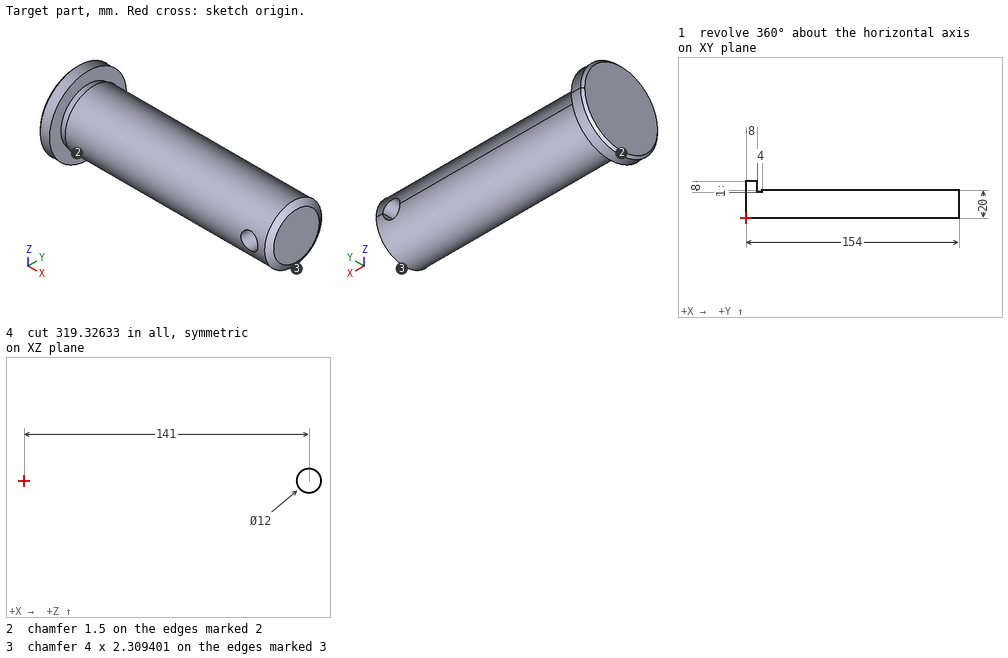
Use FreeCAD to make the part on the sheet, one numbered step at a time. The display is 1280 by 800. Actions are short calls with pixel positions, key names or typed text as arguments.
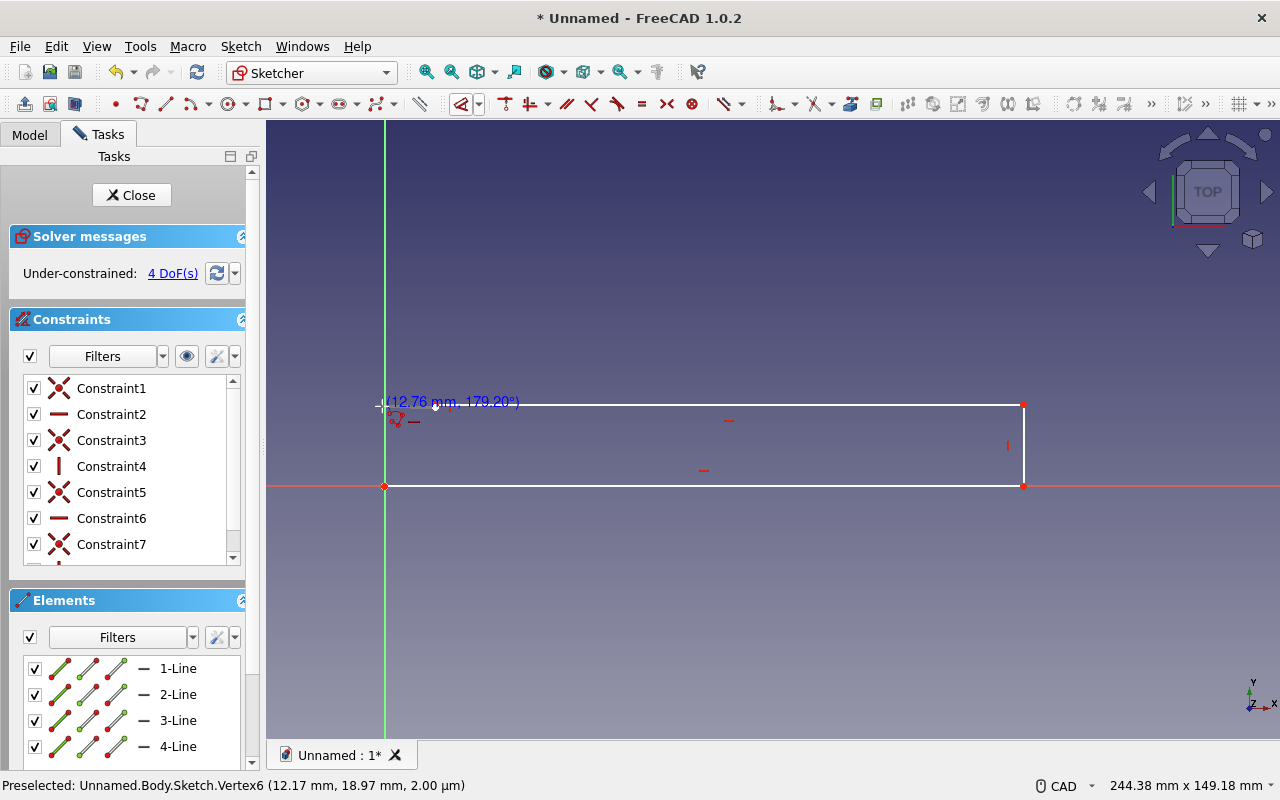
click(418, 407)
click(418, 374)
click(394, 374)
click(385, 486)
key(Escape)
key(Escape)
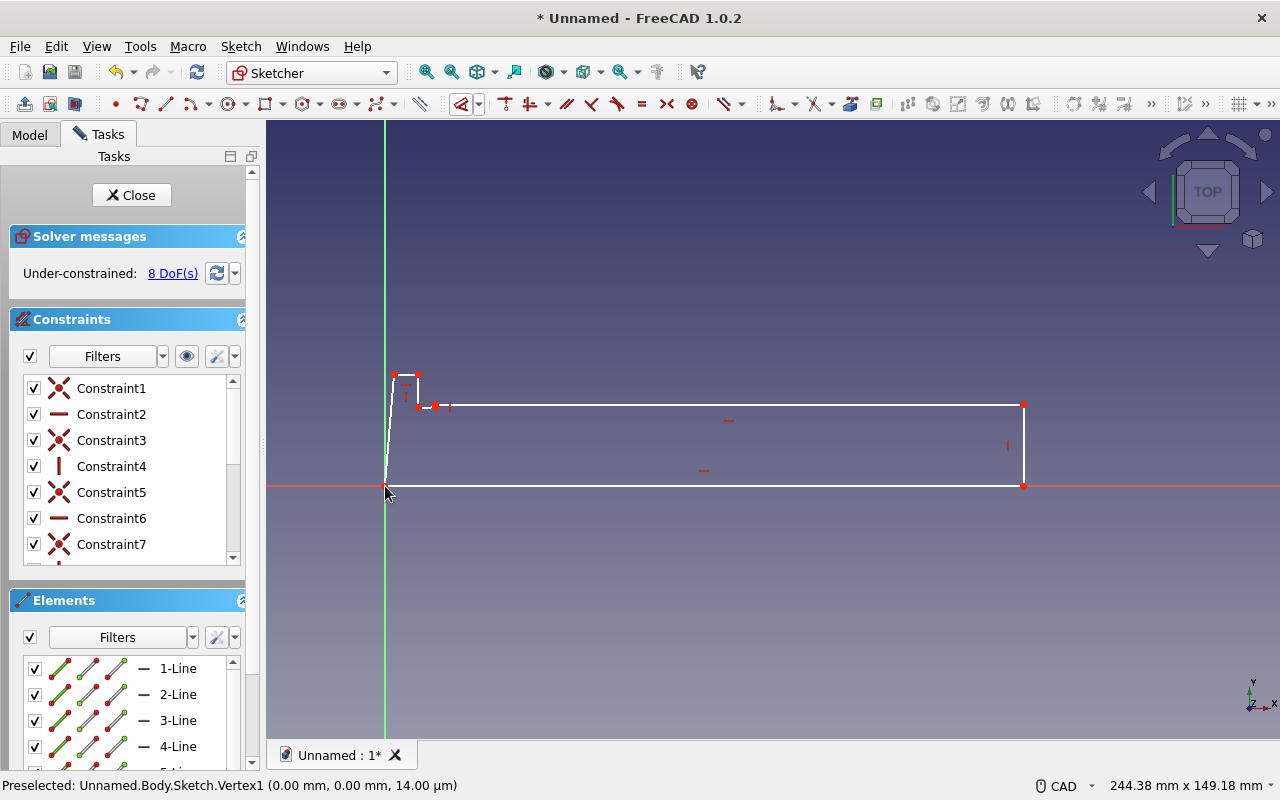
scroll(427, 408, up, 3)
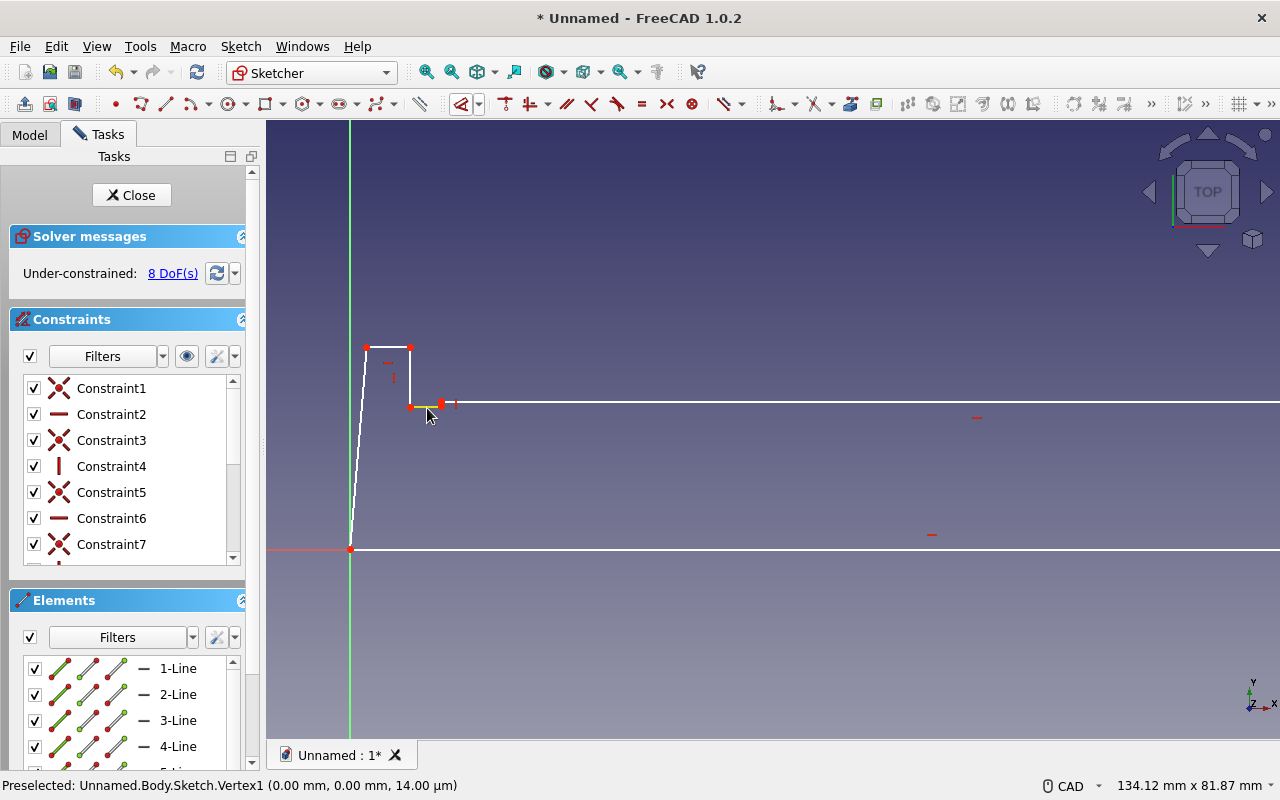
click(426, 407)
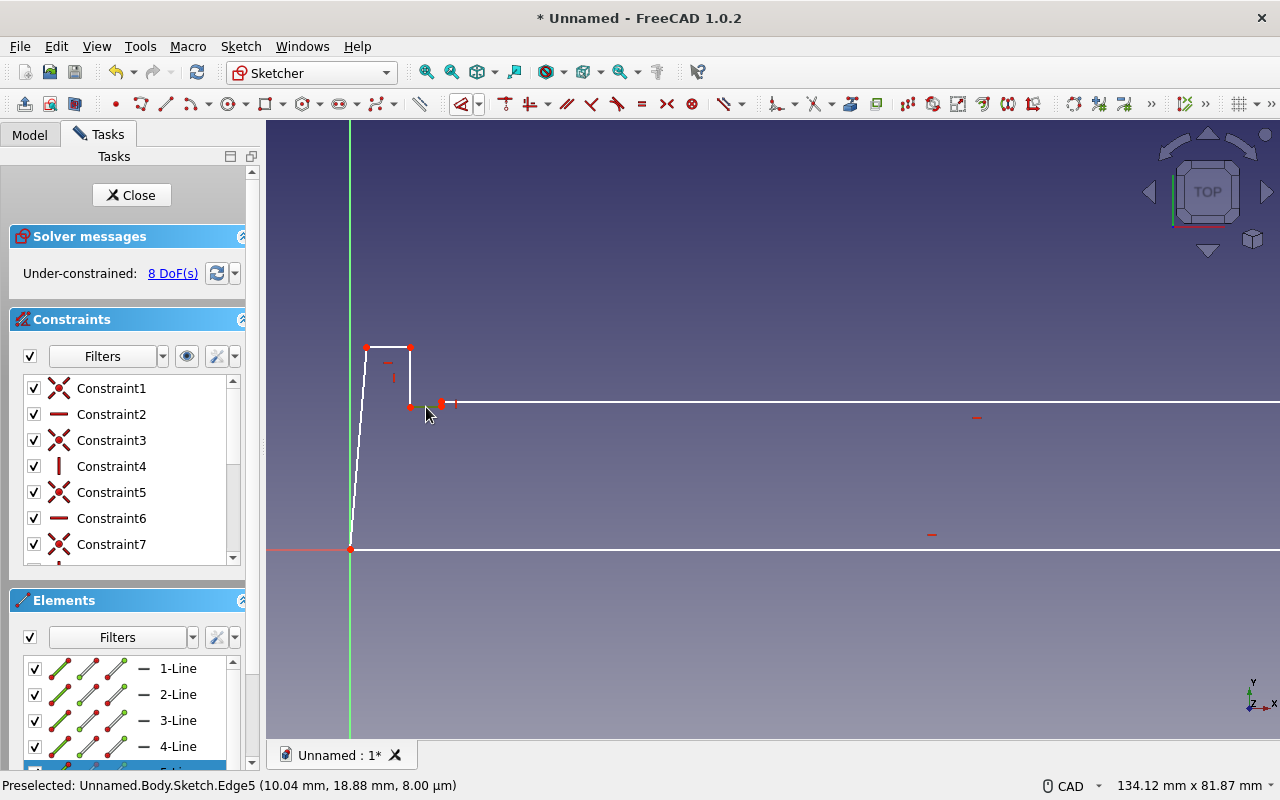
key(h)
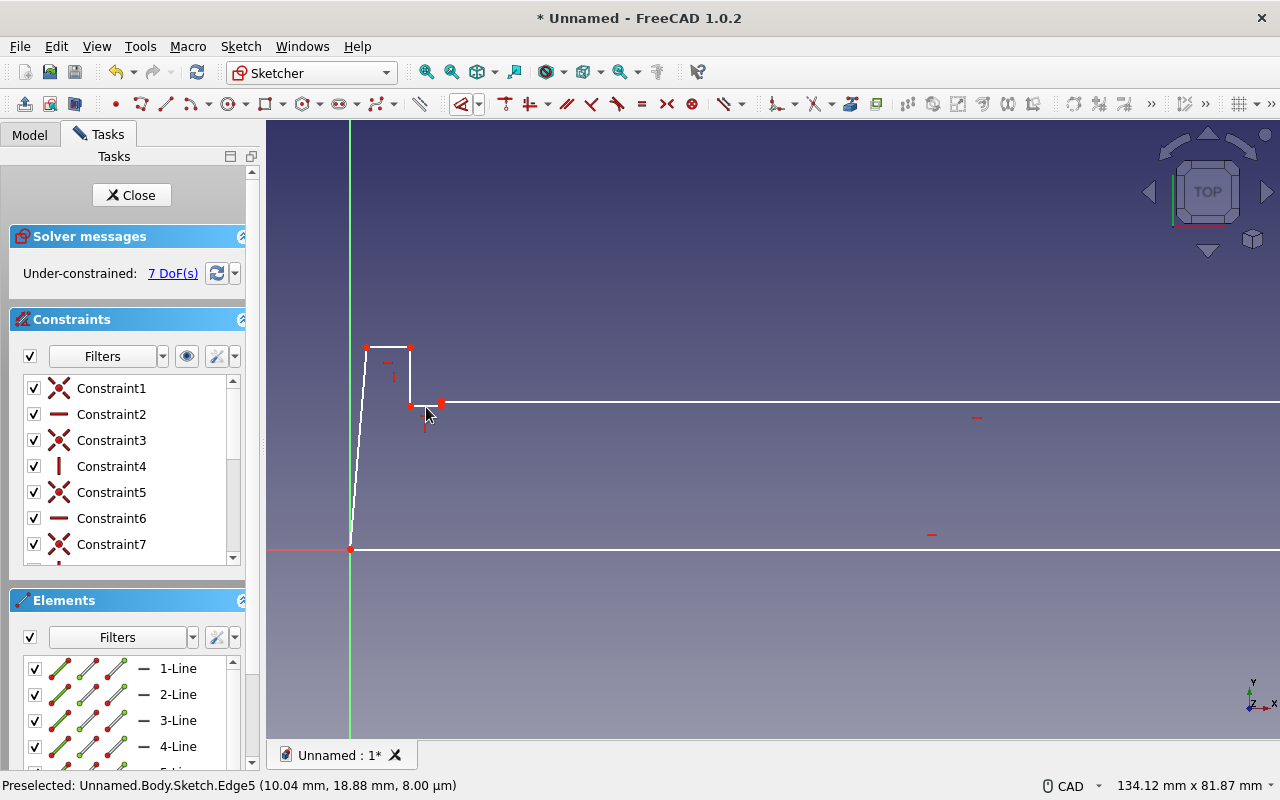
click(362, 408)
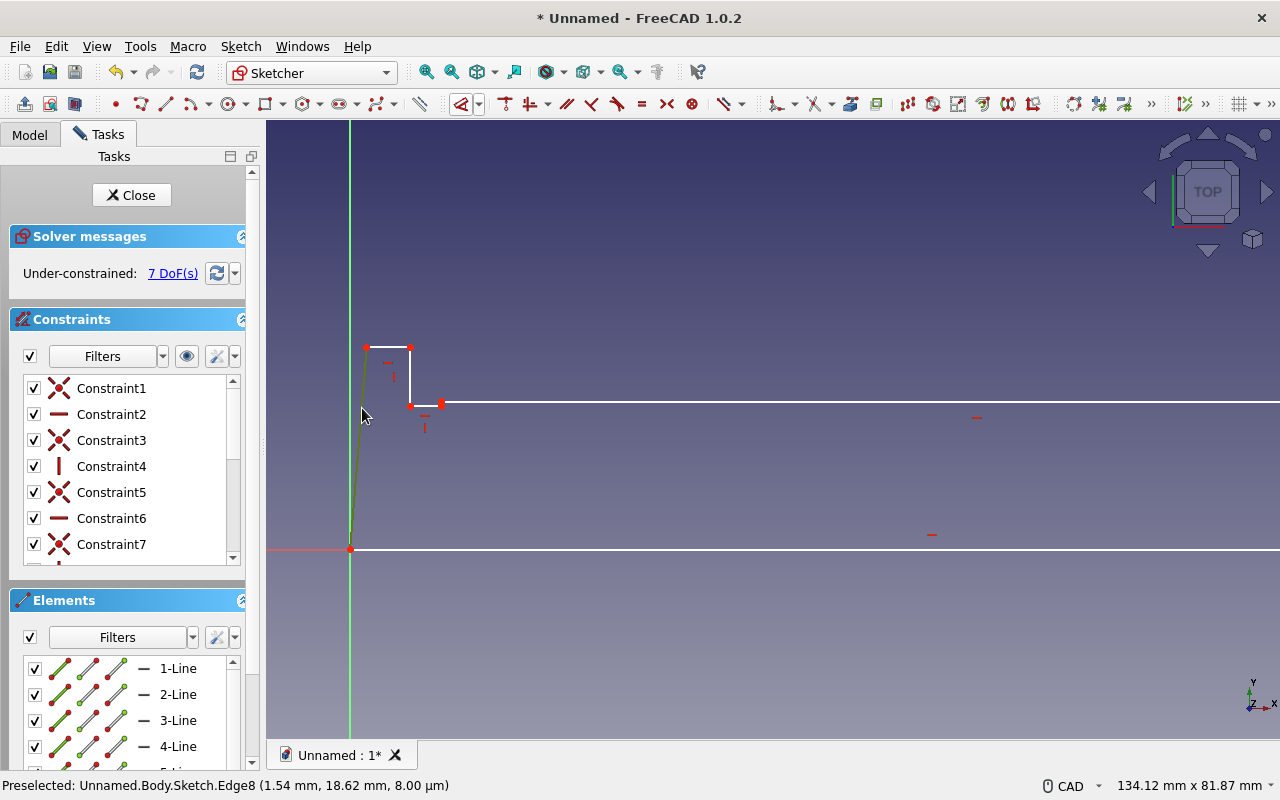
click(548, 104)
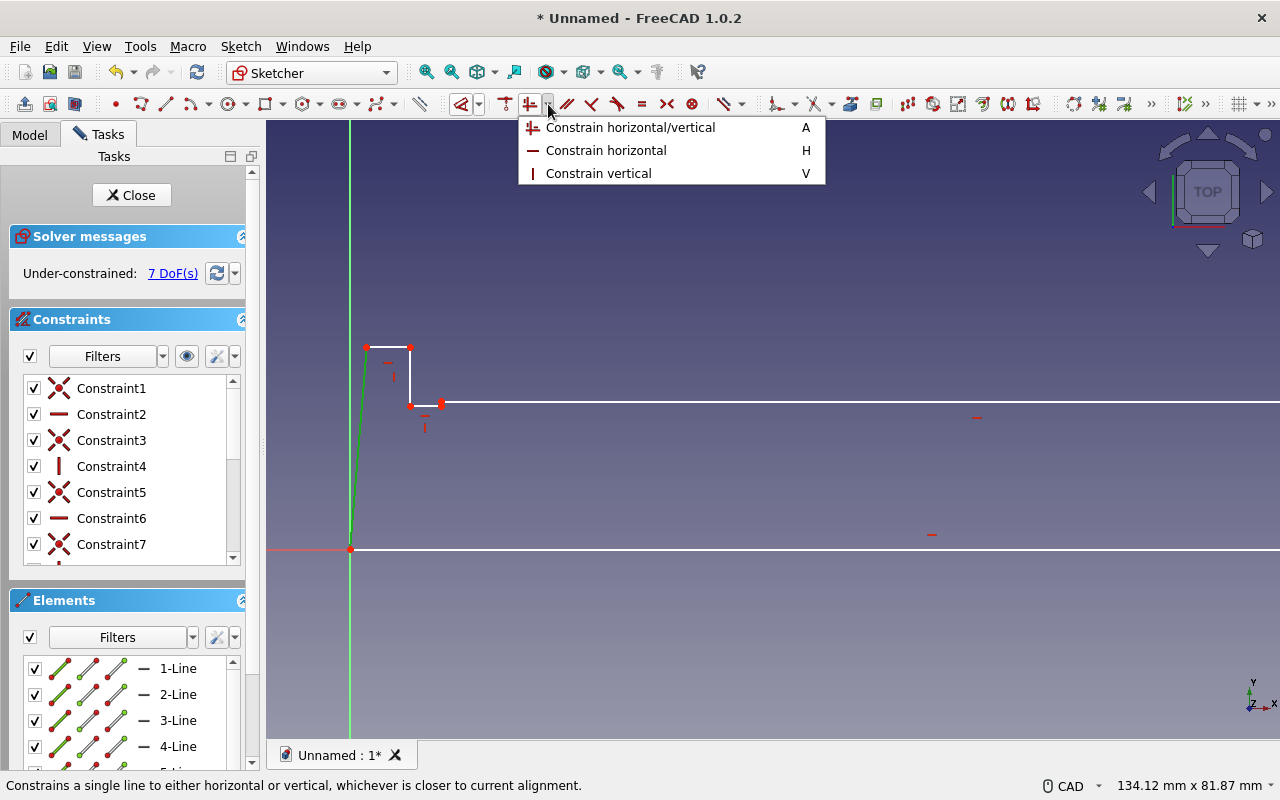
click(672, 174)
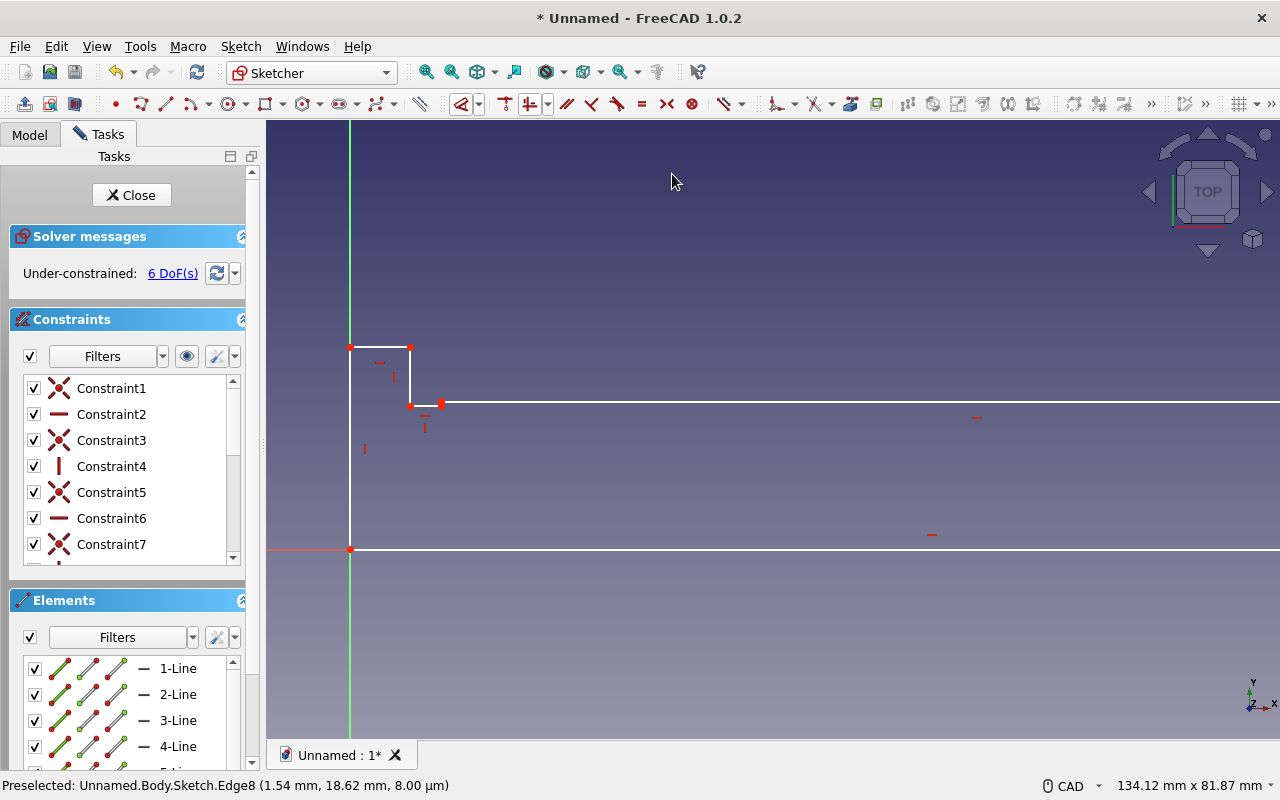
scroll(442, 404, up, 9)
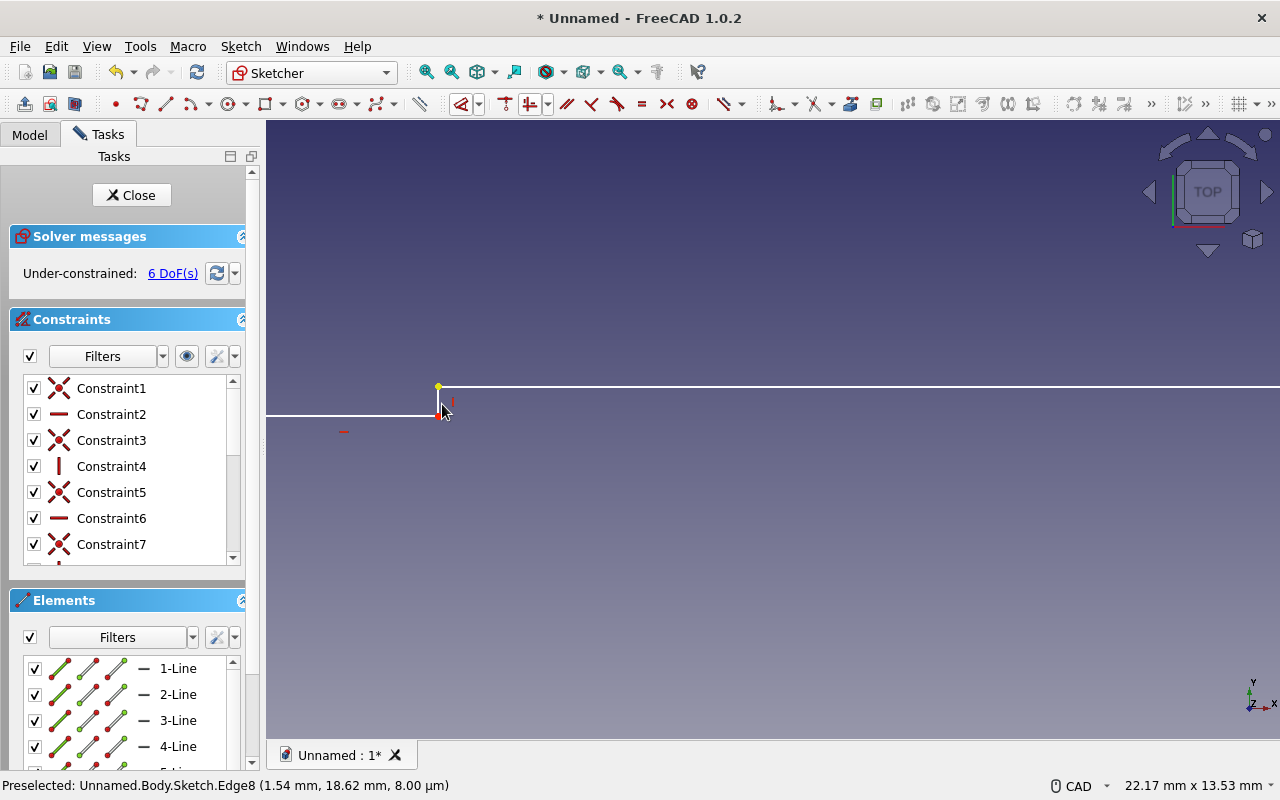
click(438, 402)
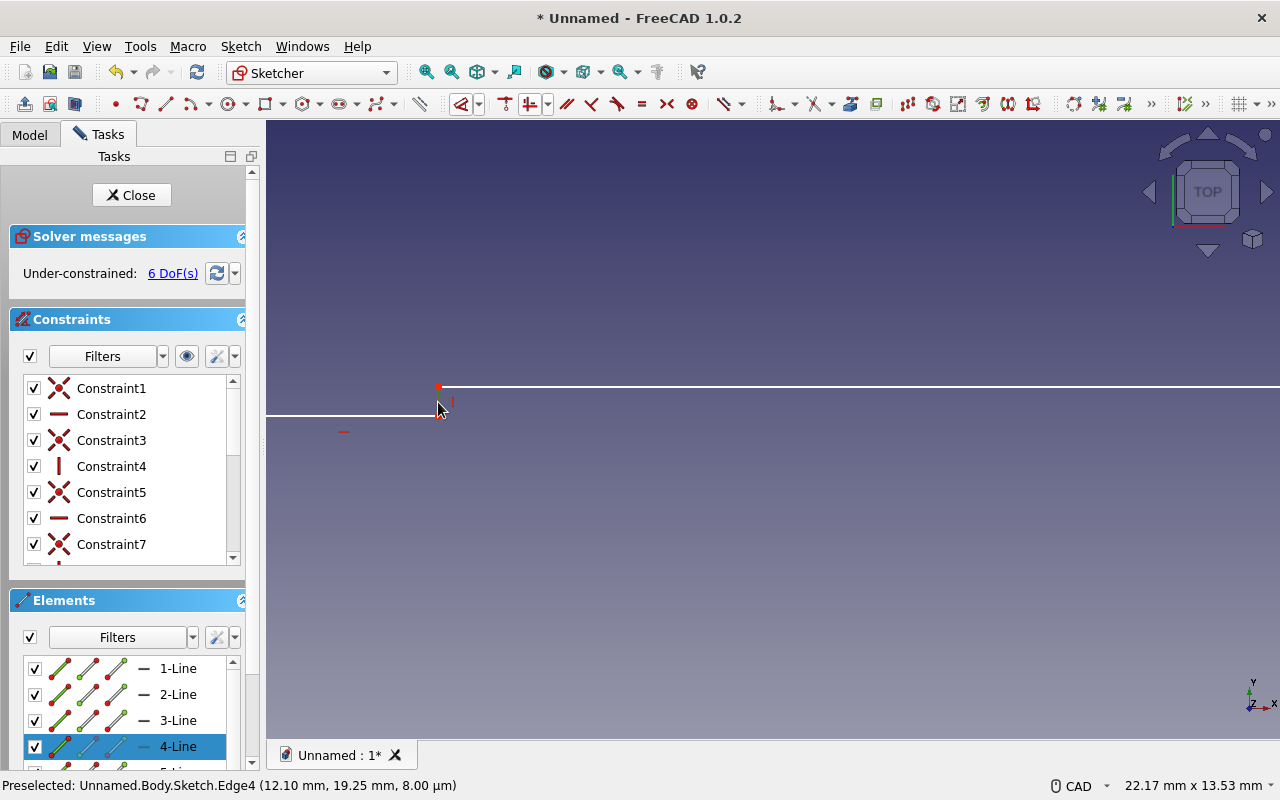
key(i)